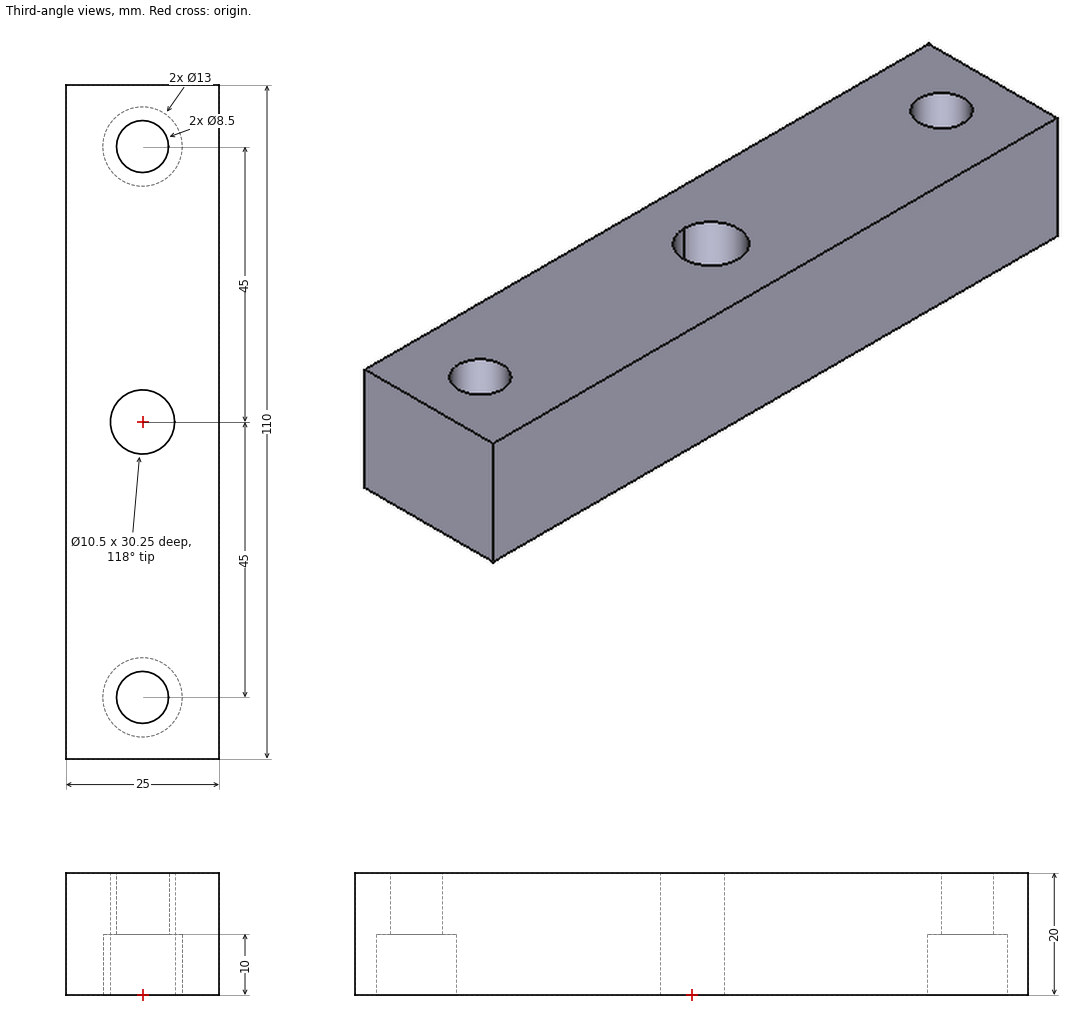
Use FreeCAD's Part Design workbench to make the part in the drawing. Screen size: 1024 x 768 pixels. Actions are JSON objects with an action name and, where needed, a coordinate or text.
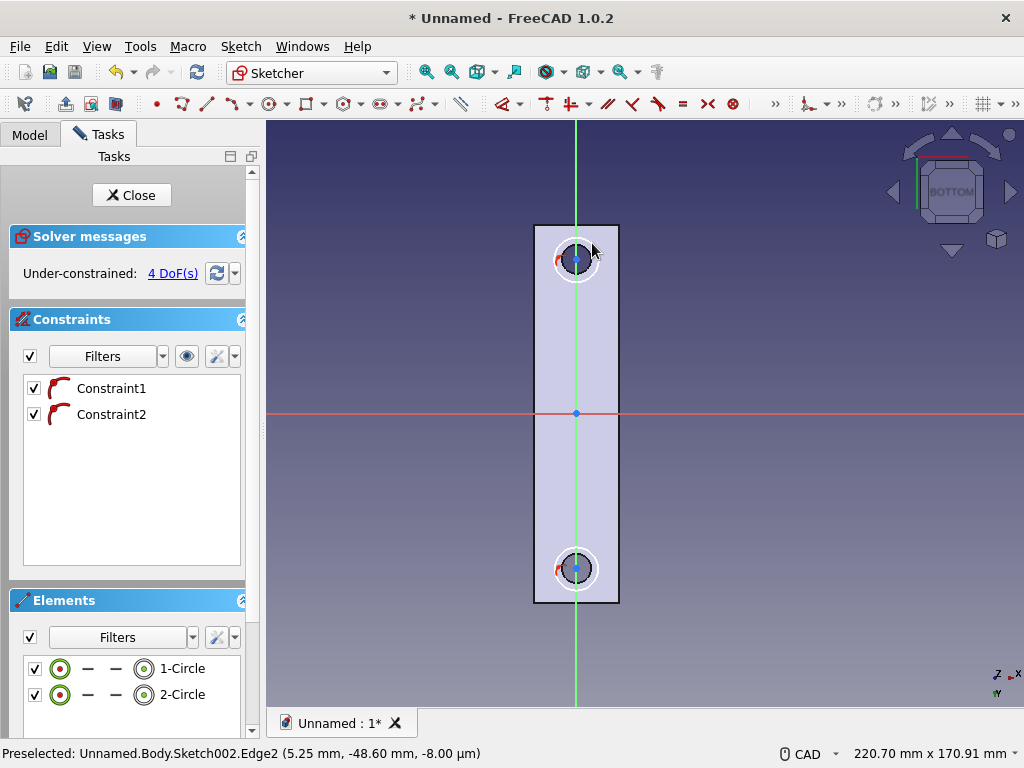
{"action": "left_click", "coordinate": [592, 554]}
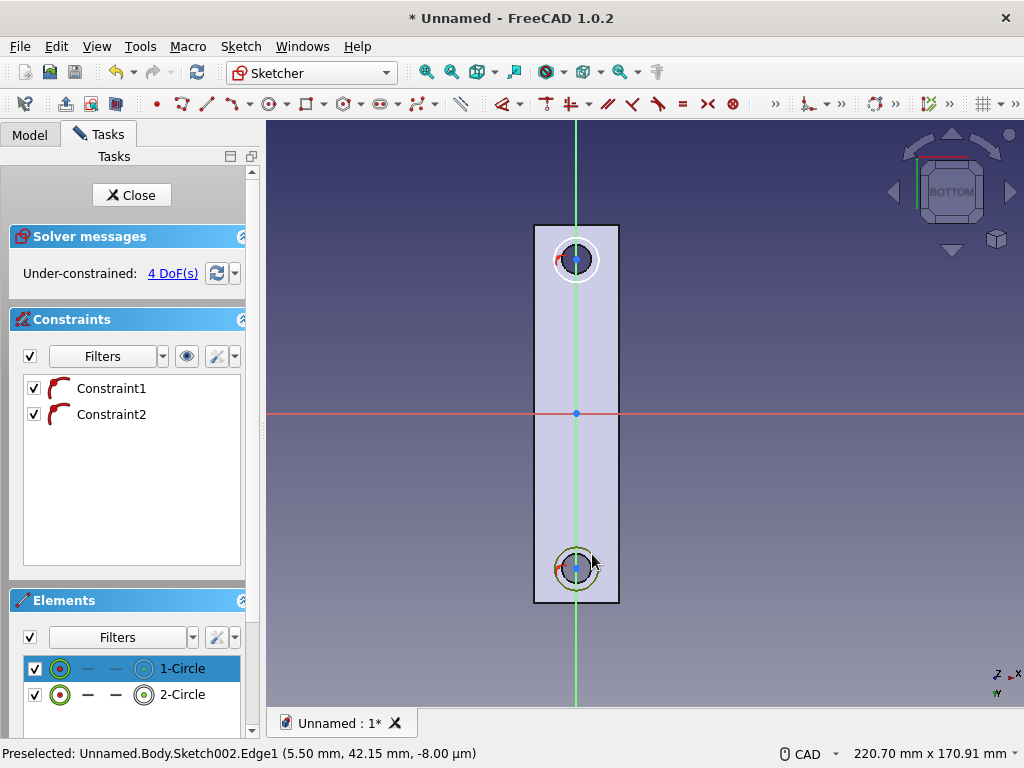
{"action": "left_click", "coordinate": [592, 244]}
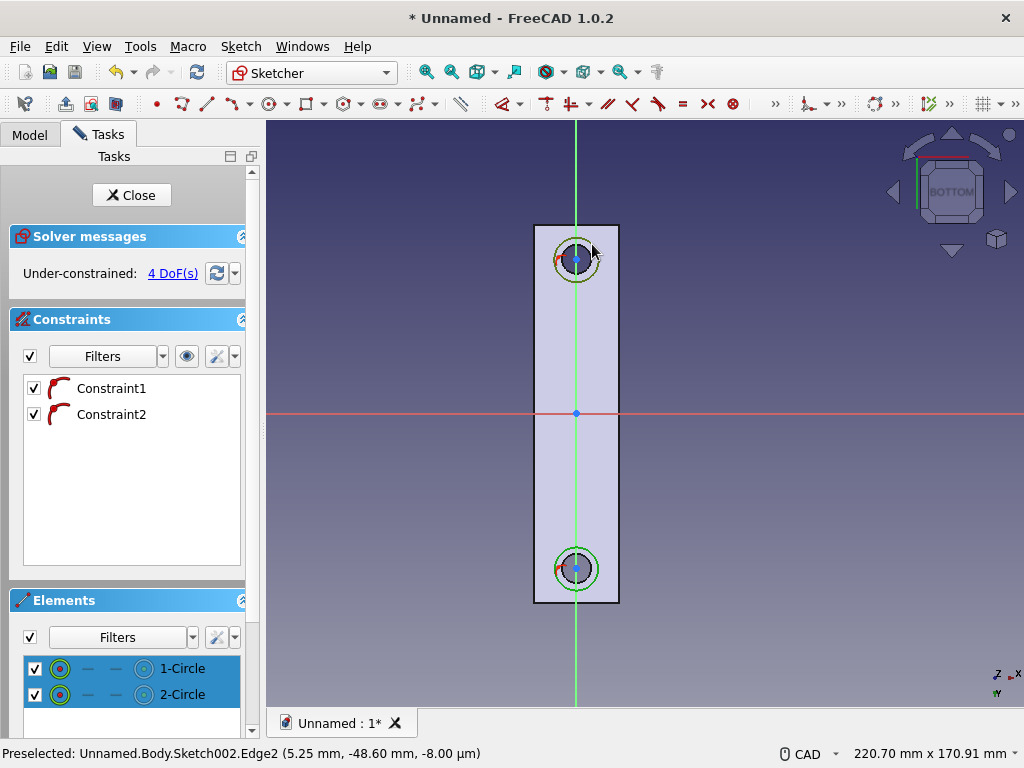
{"action": "key", "text": "e"}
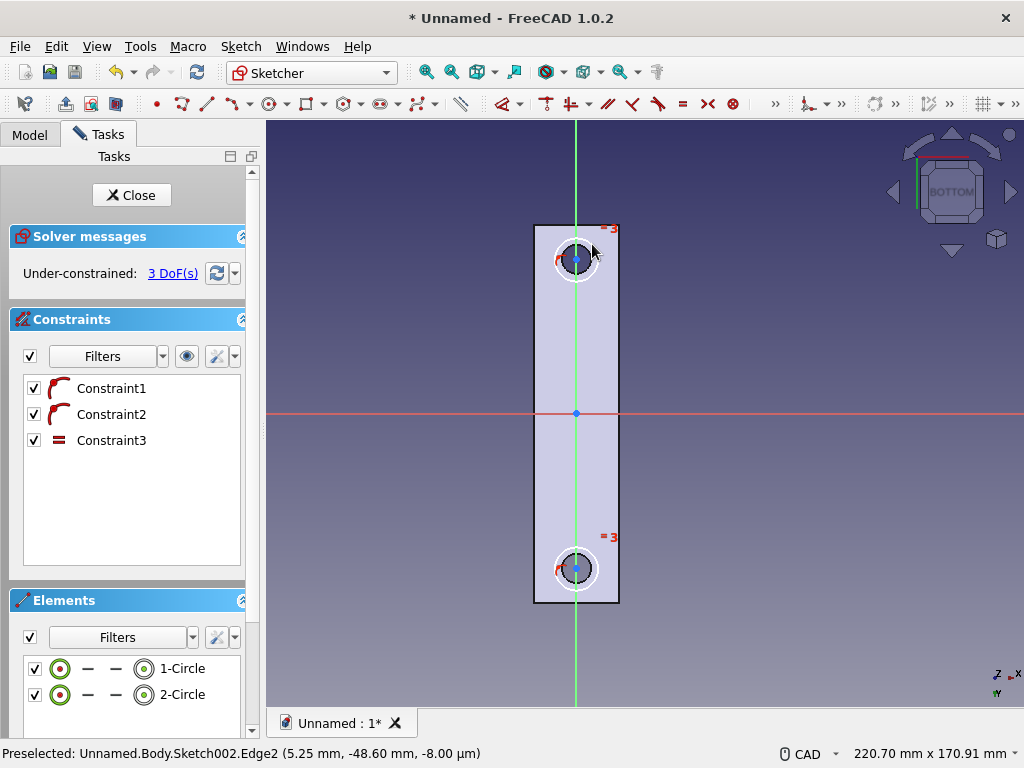
{"action": "left_click", "coordinate": [502, 104]}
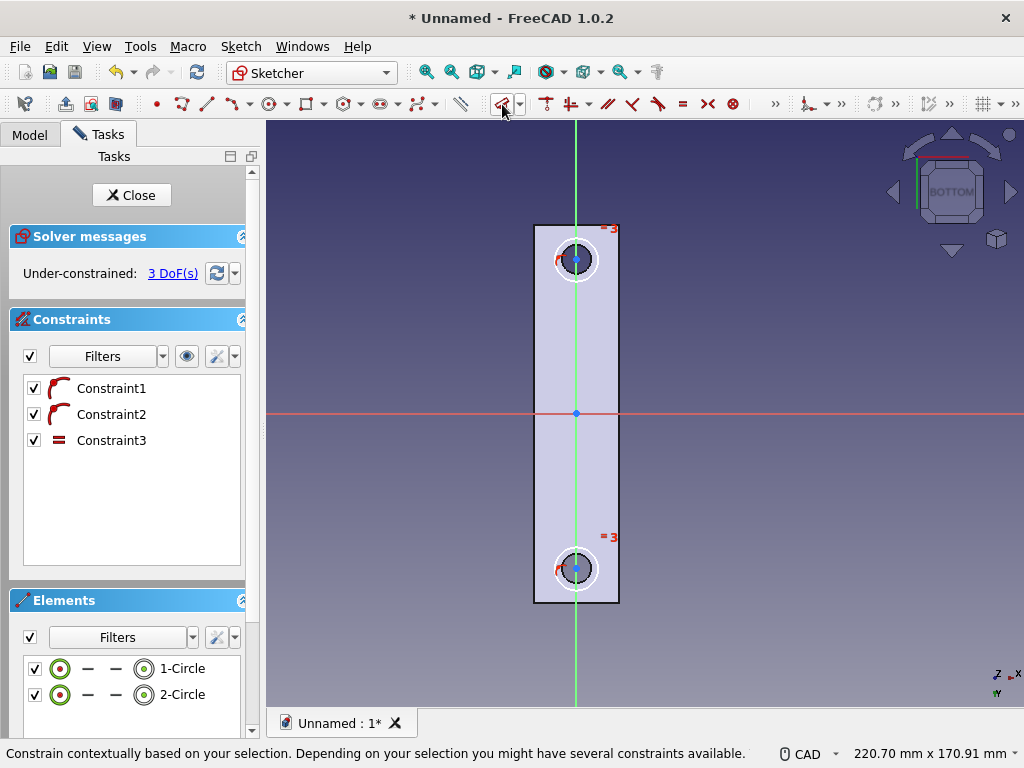
{"action": "left_click", "coordinate": [592, 554]}
{"action": "left_click", "coordinate": [615, 532]}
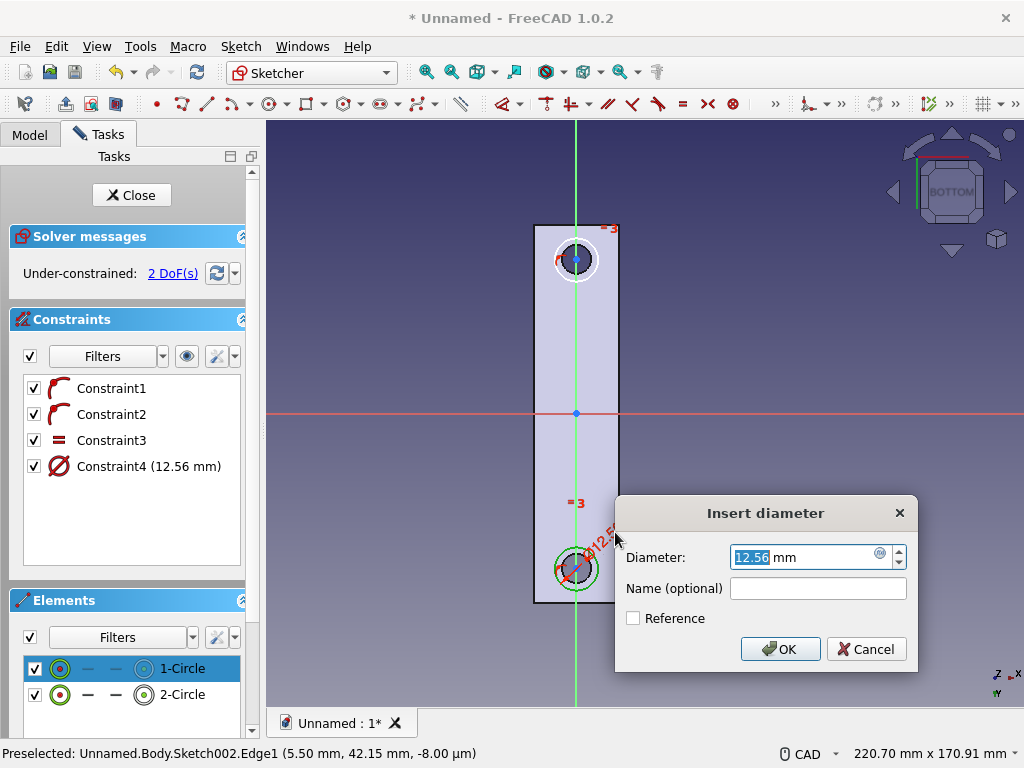
{"action": "type", "text": "13"}
{"action": "key", "text": "Return"}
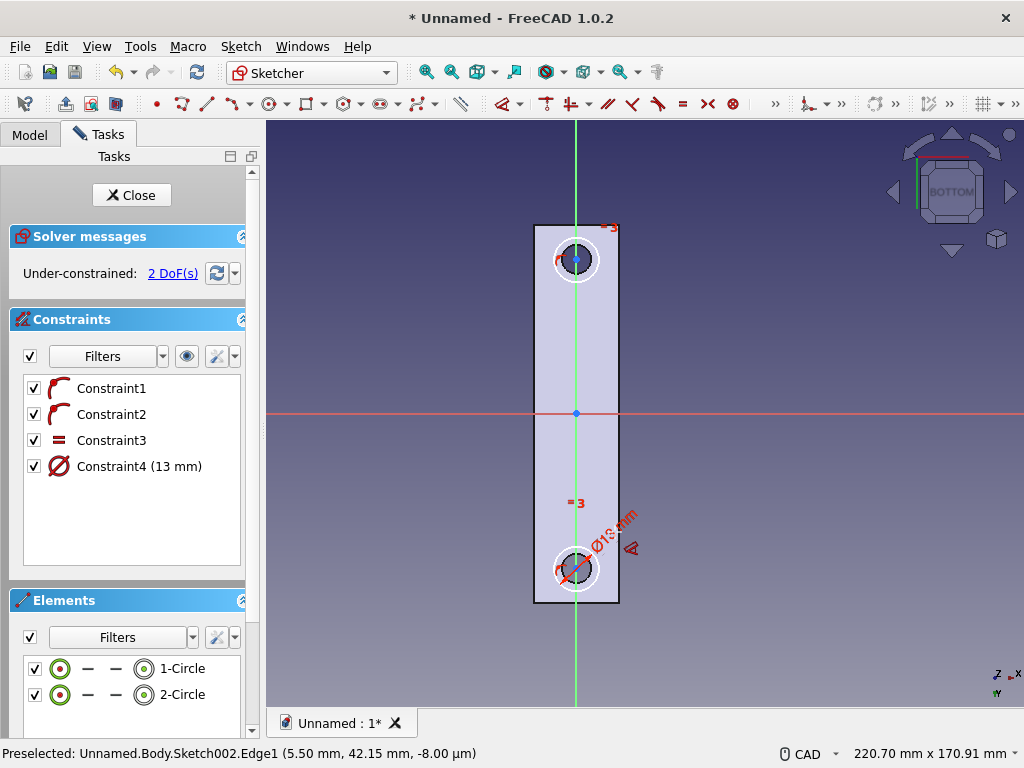
{"action": "left_click", "coordinate": [577, 569]}
{"action": "left_click", "coordinate": [611, 491]}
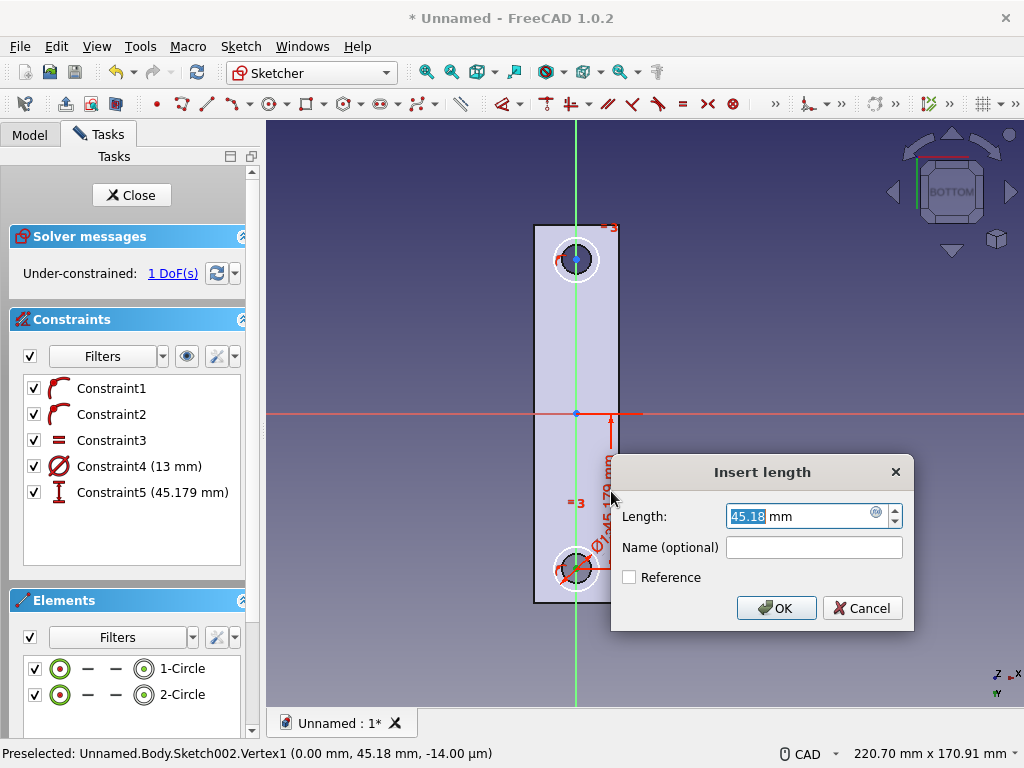
{"action": "type", "text": "45"}
{"action": "key", "text": "Return"}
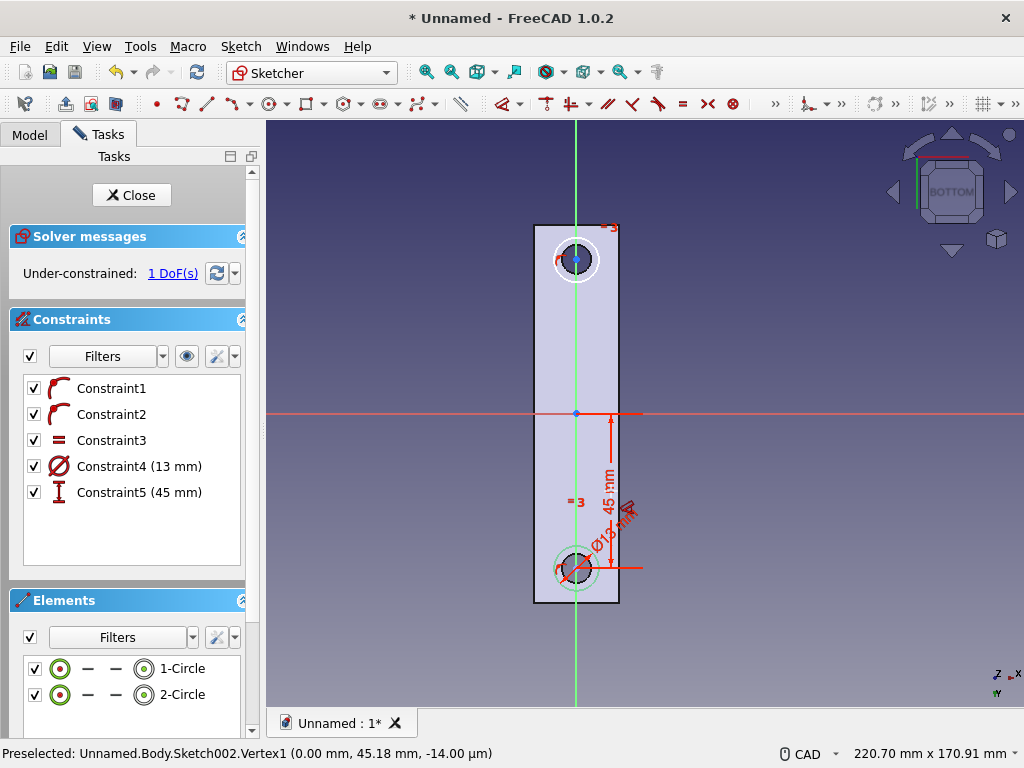
{"action": "left_click", "coordinate": [577, 260]}
{"action": "left_click", "coordinate": [611, 337]}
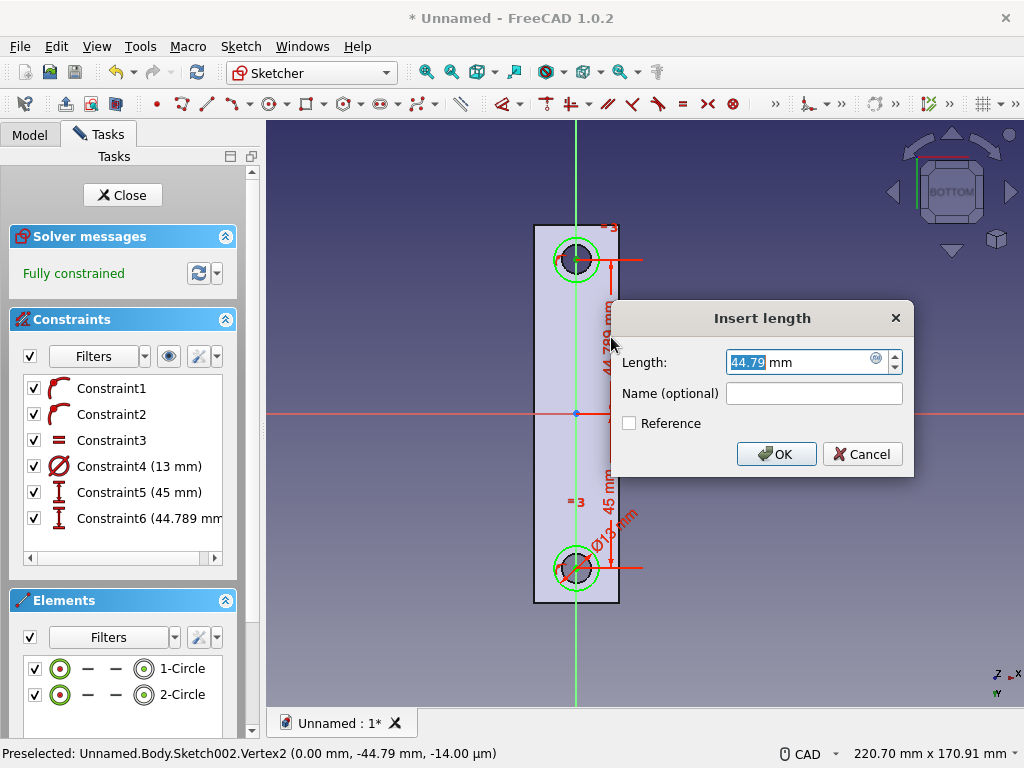
{"action": "type", "text": "45"}
{"action": "key", "text": "Return"}
{"action": "key", "text": "Escape"}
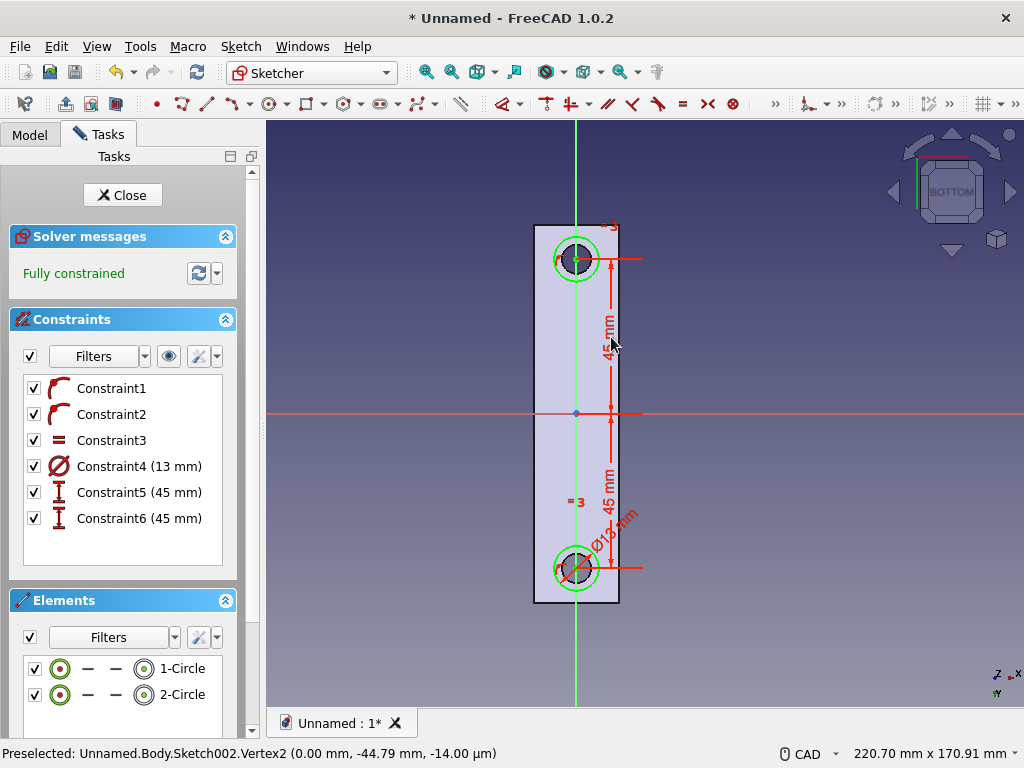
{"action": "left_click", "coordinate": [123, 195]}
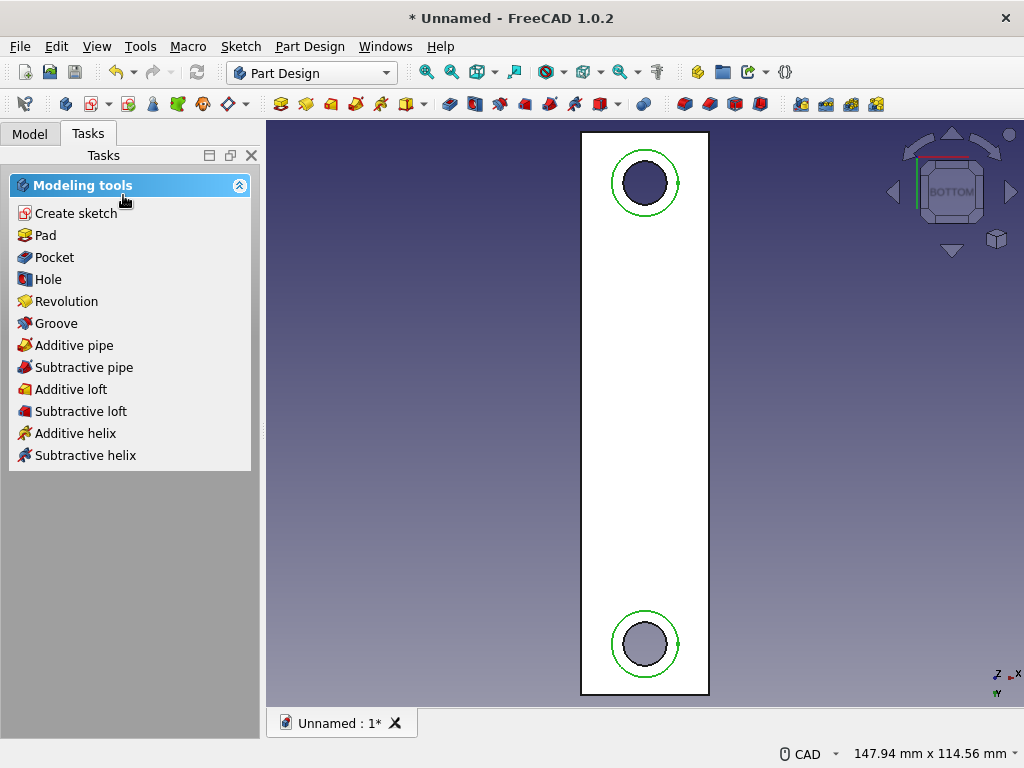
{"action": "left_click", "coordinate": [450, 104]}